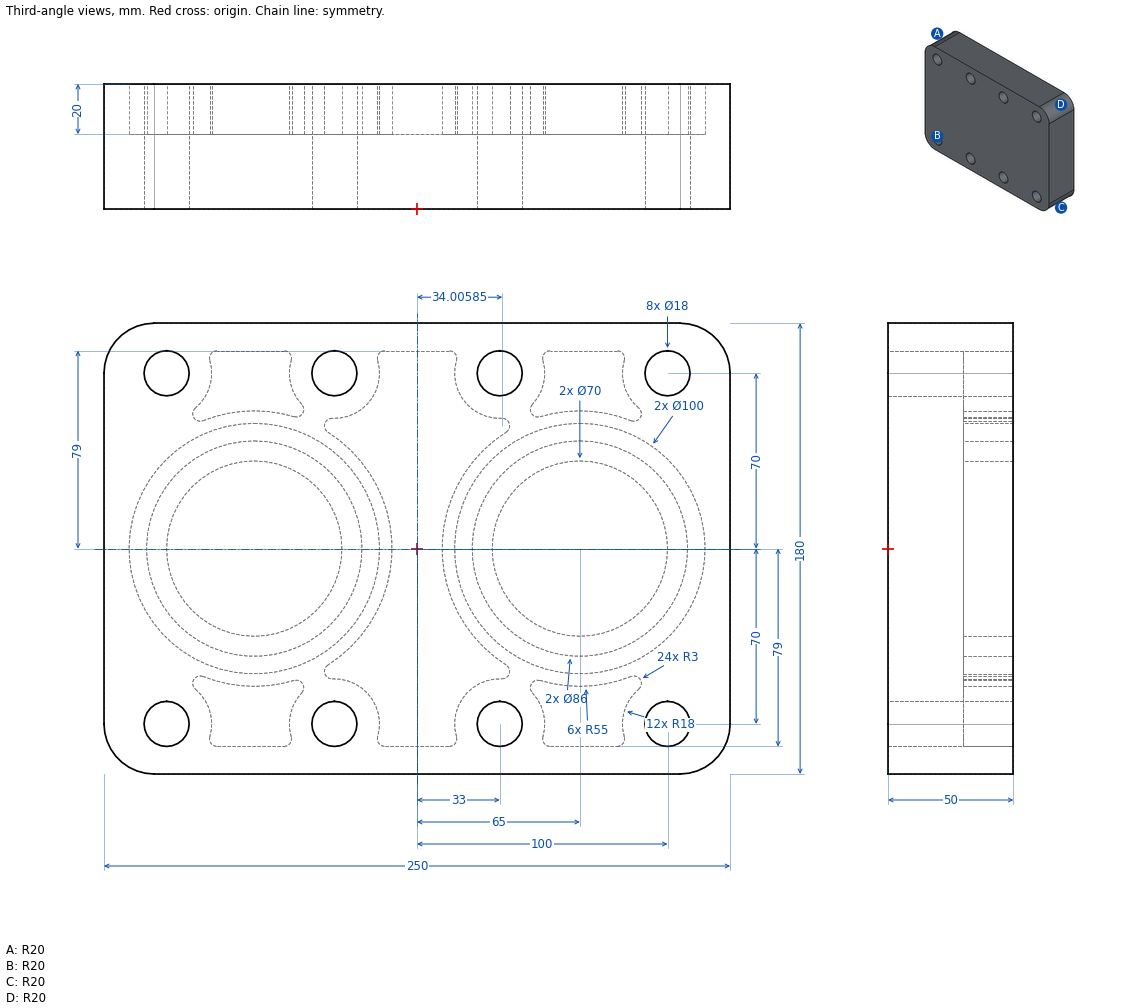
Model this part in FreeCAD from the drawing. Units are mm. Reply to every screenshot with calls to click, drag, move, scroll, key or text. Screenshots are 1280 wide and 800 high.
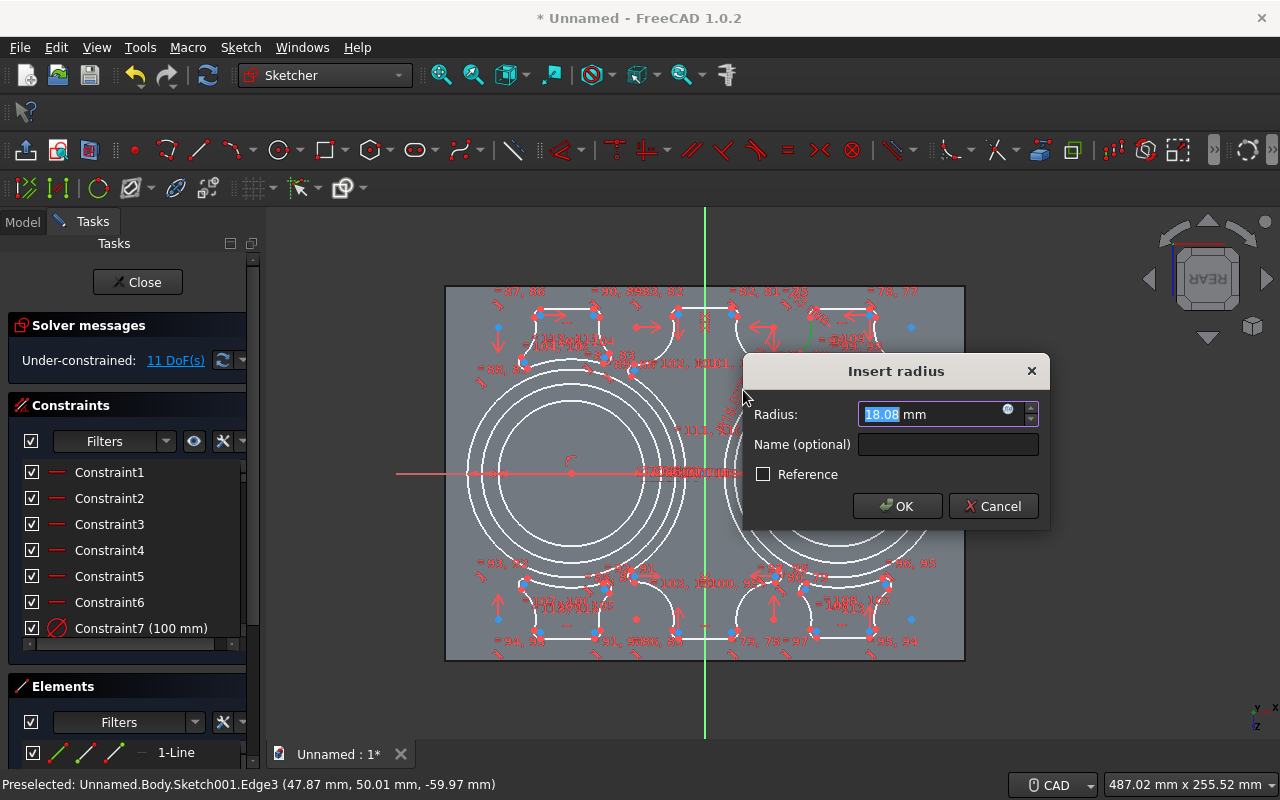
text(18)
key(Return)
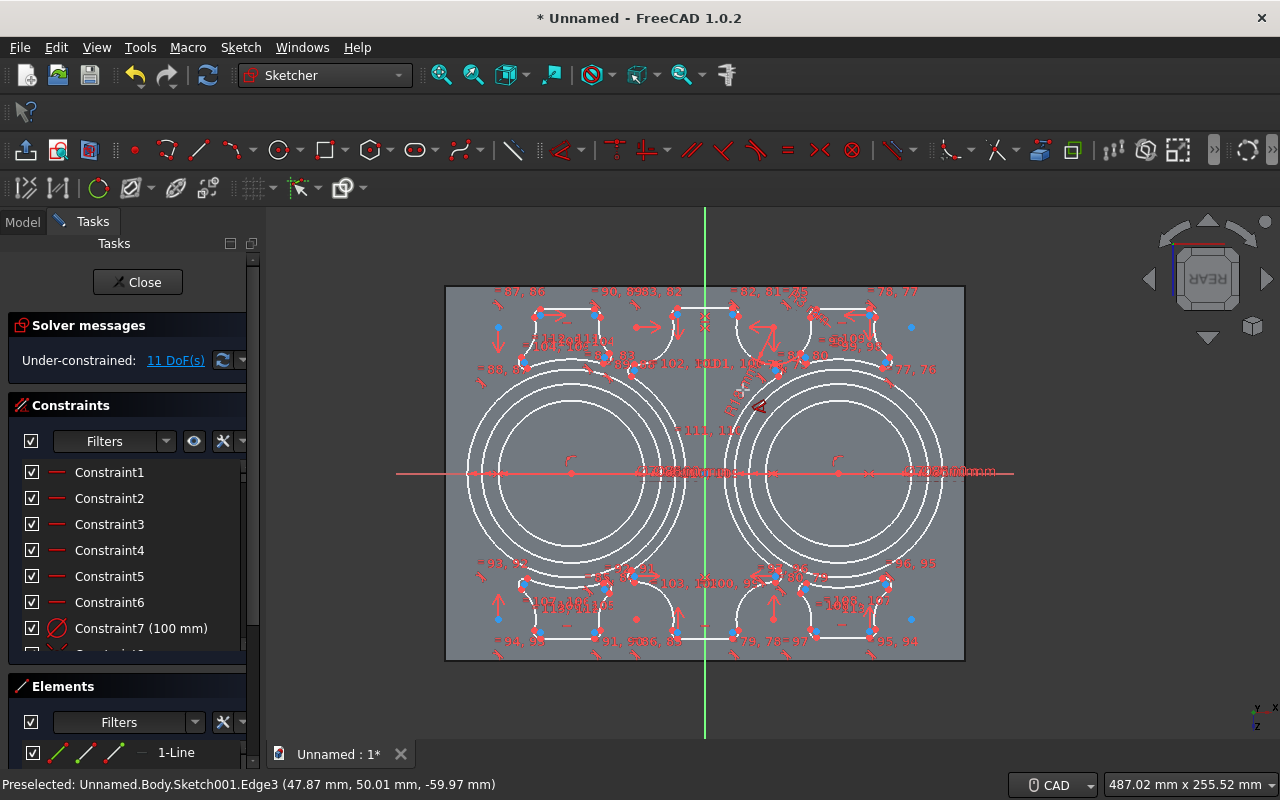
scroll(861, 362, up, 2)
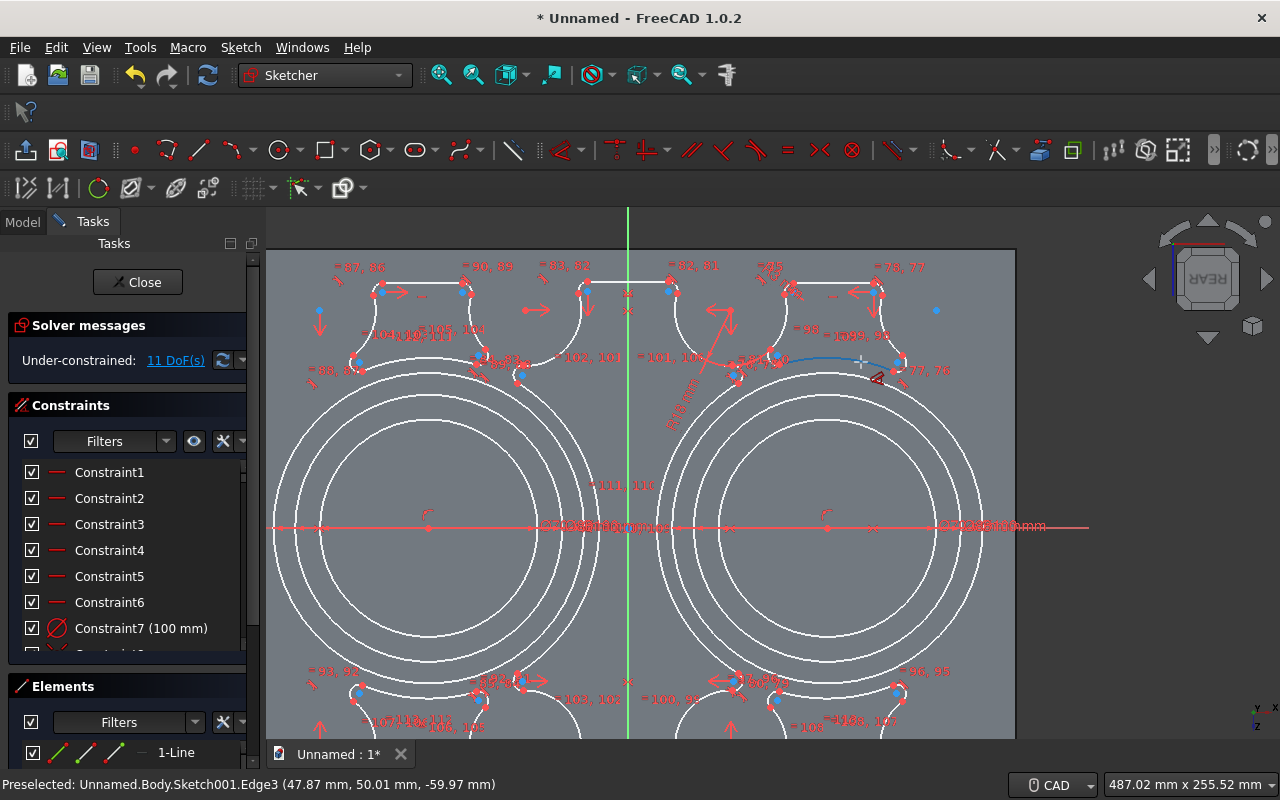
click(860, 361)
click(866, 330)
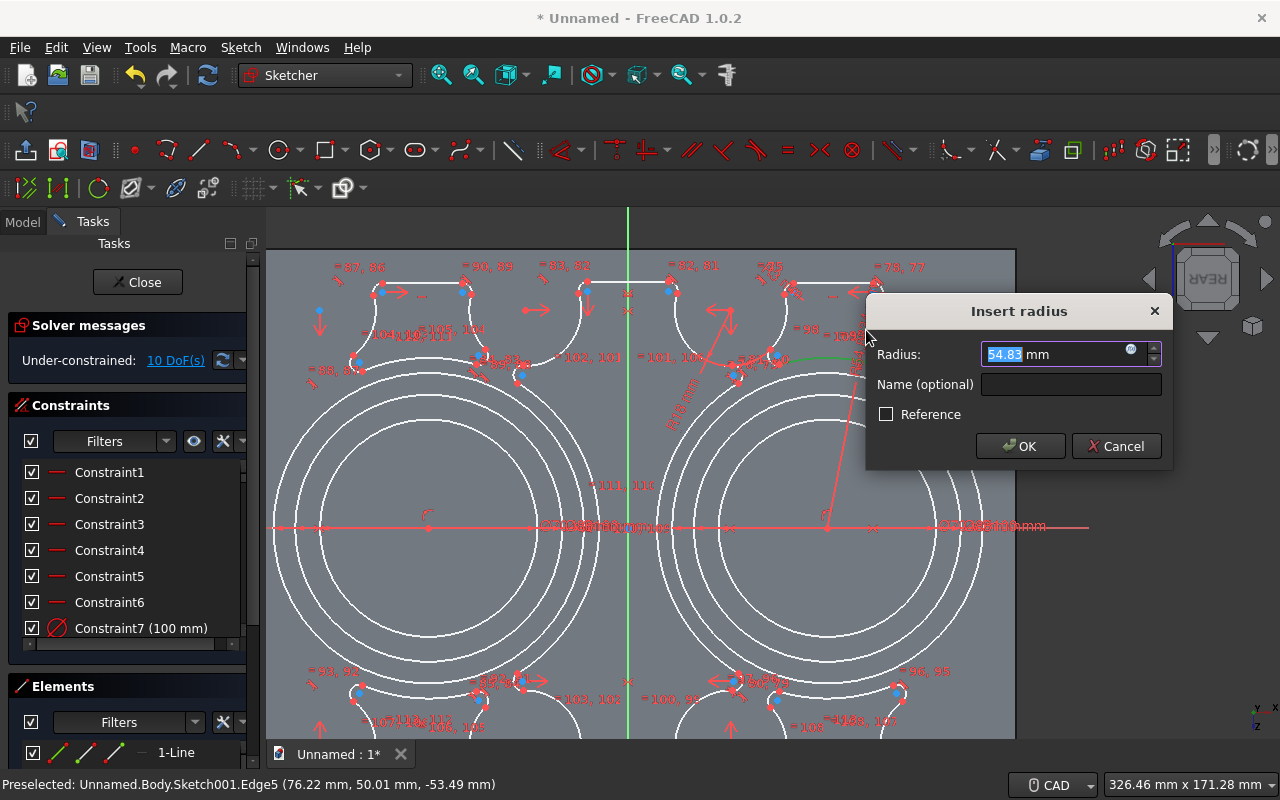
text(55)
key(Return)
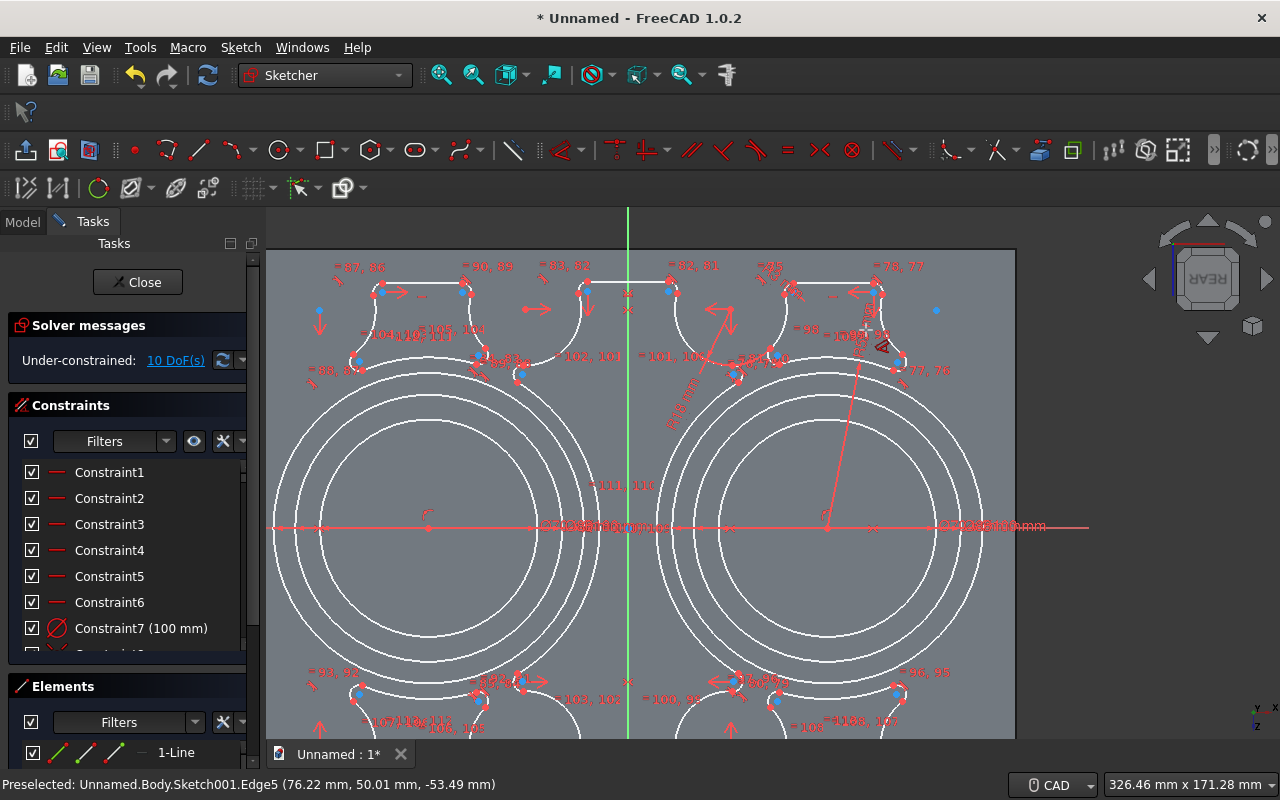
click(827, 528)
click(774, 562)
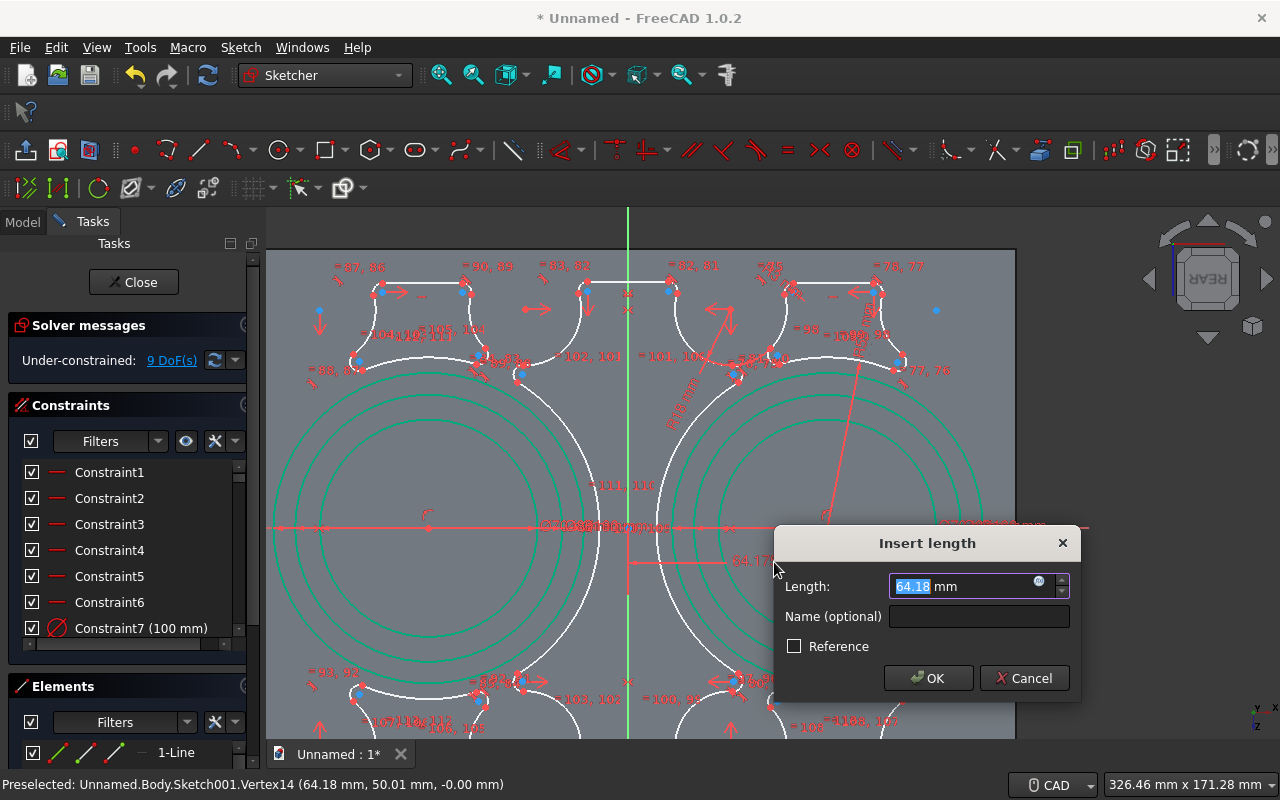
text(65)
key(Return)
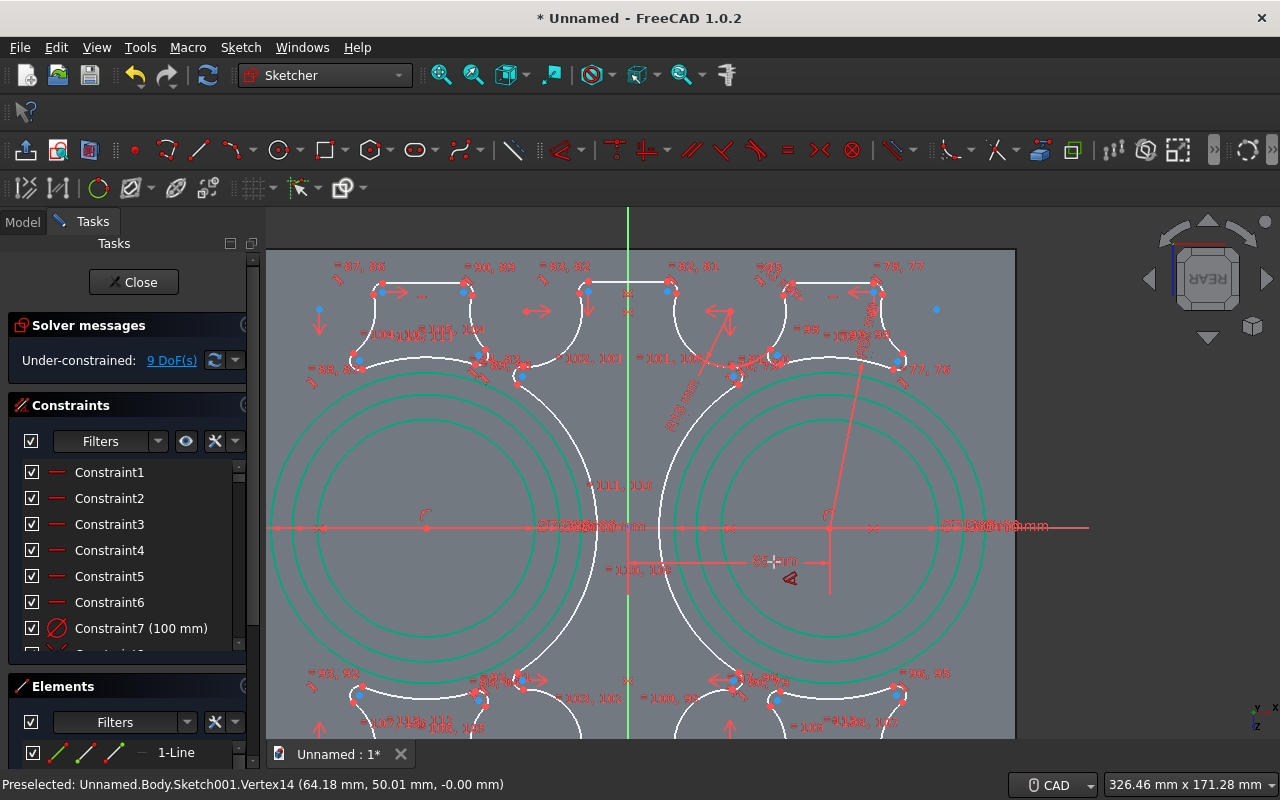
scroll(874, 283, up, 2)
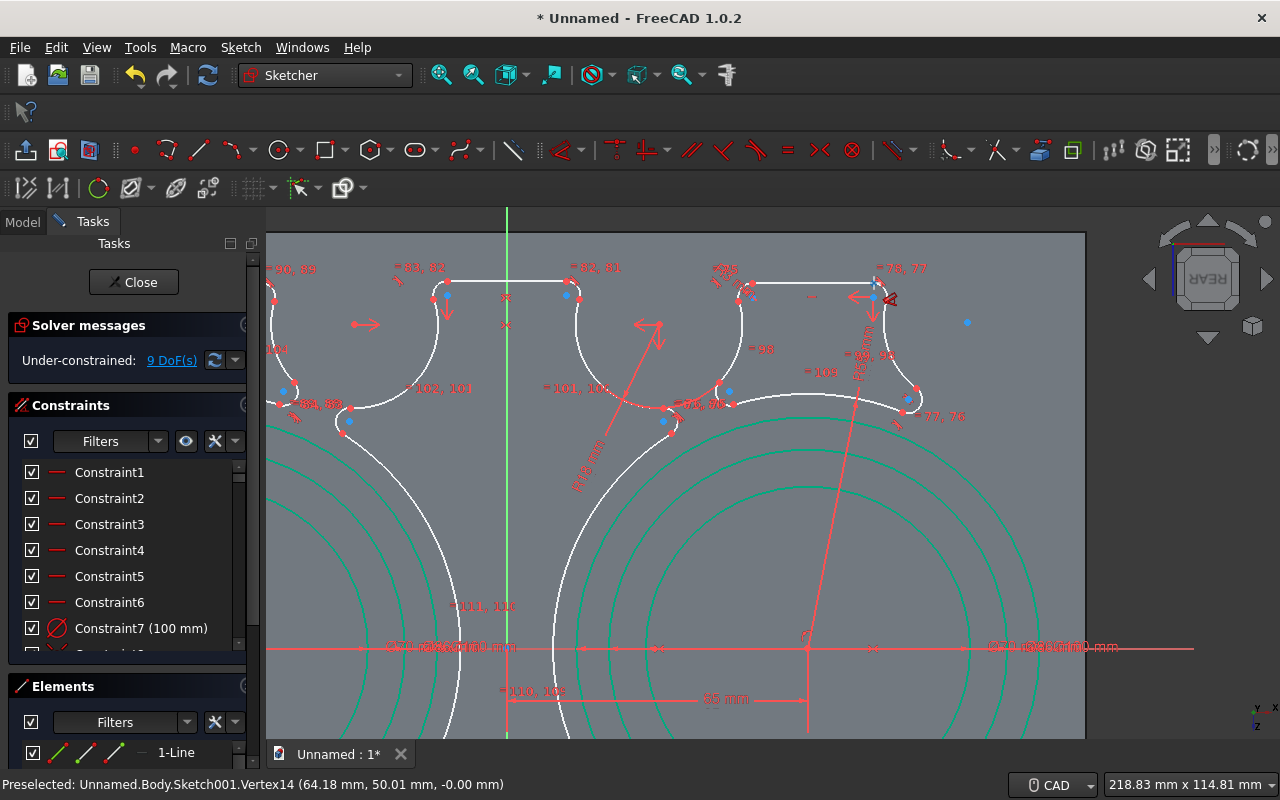
click(873, 283)
click(907, 550)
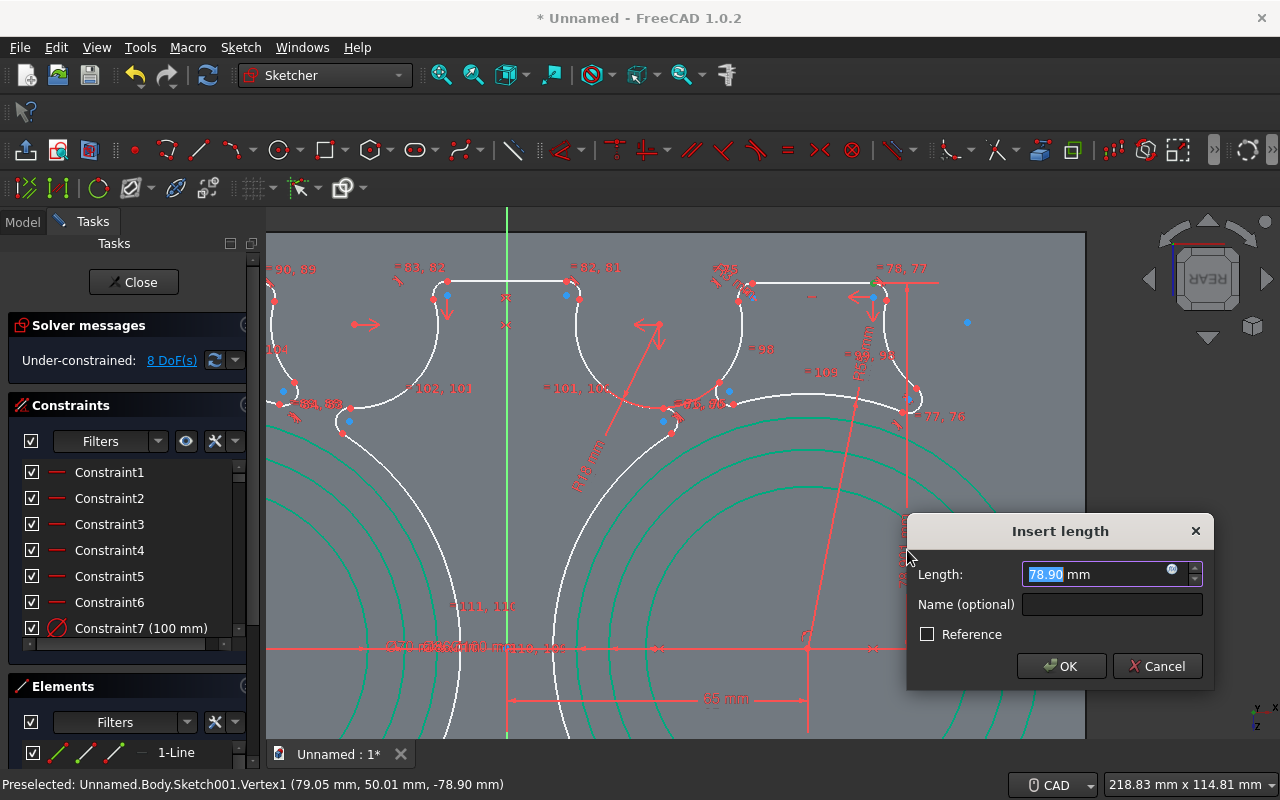
text(79)
key(Return)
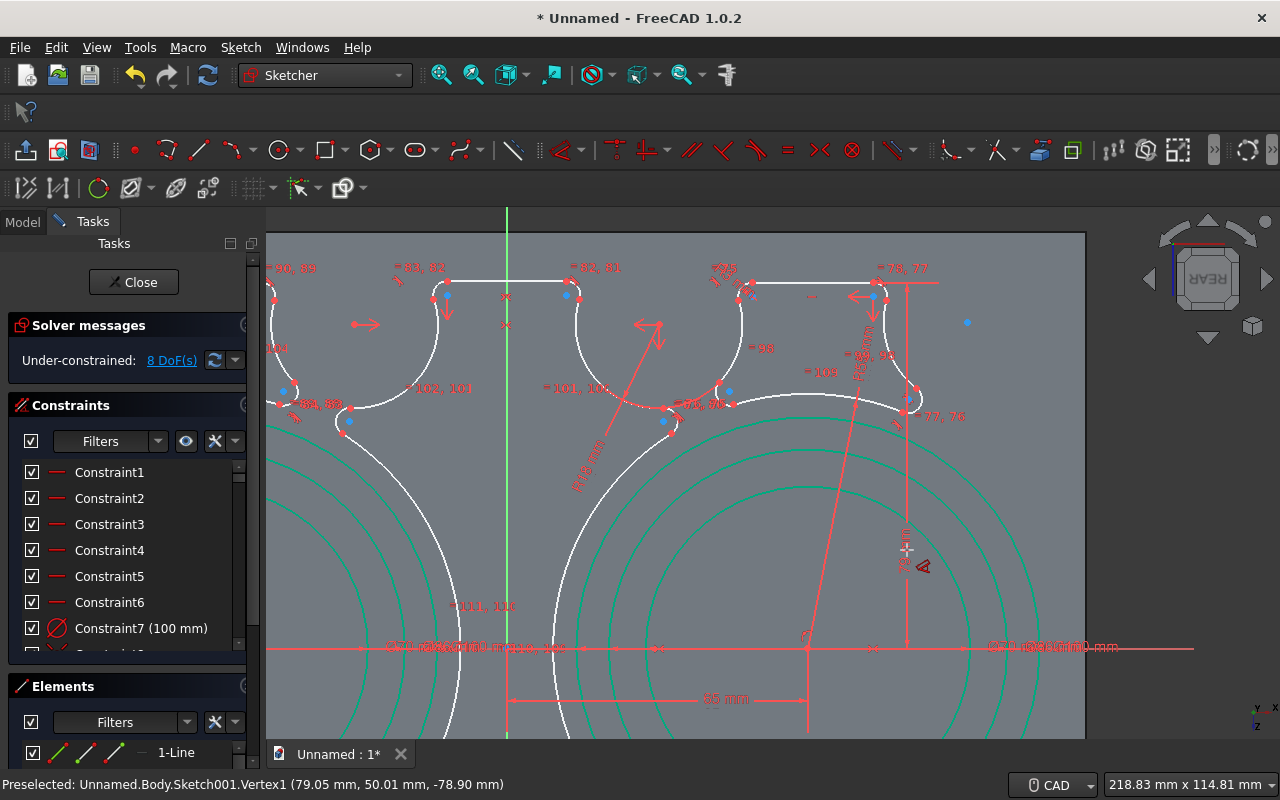
scroll(866, 330, down, 4)